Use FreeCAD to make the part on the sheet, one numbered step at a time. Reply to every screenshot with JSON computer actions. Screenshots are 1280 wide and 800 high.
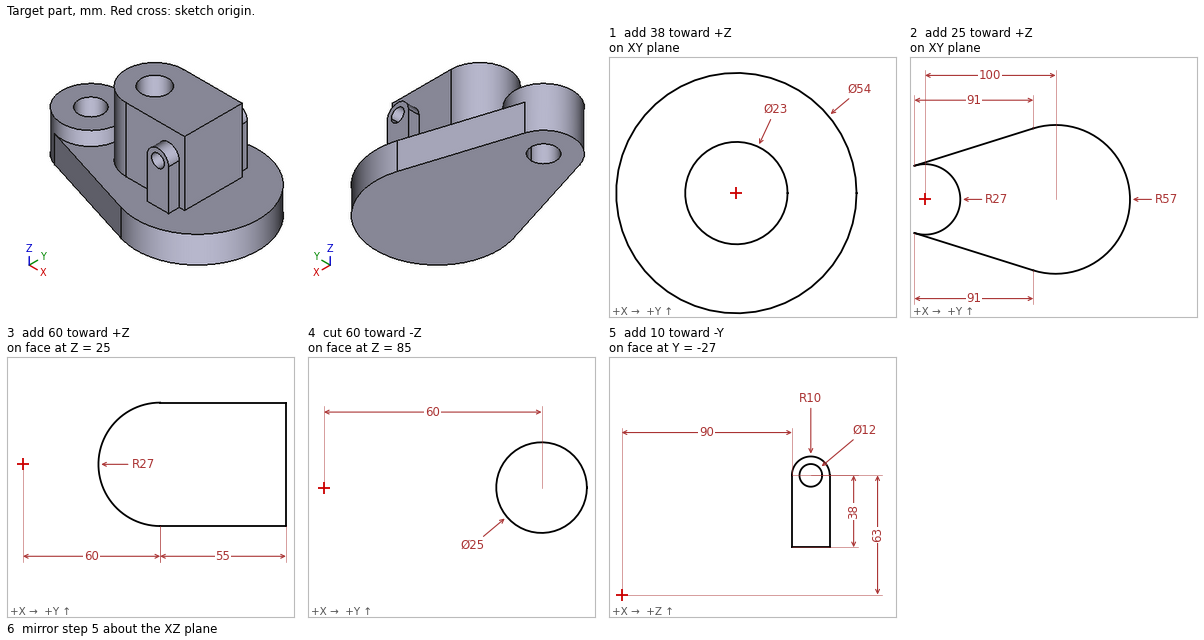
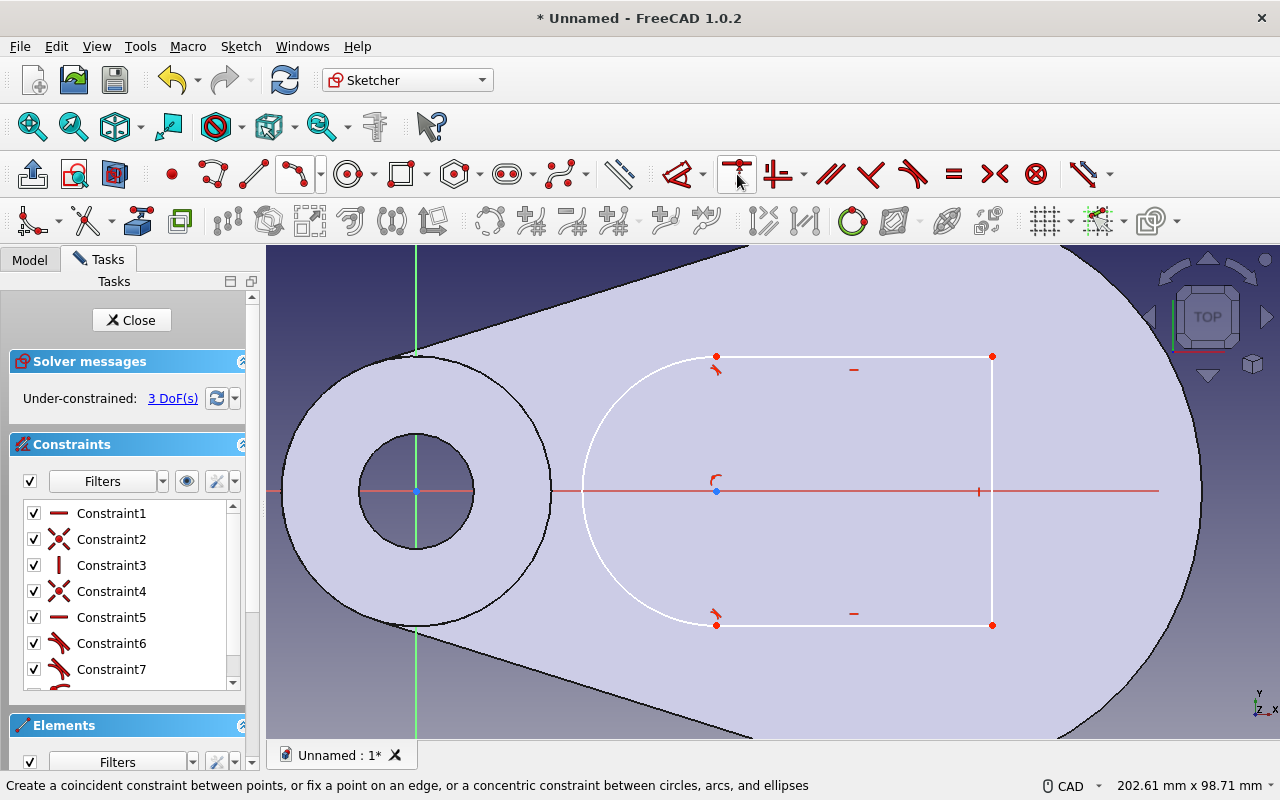
{"action": "left_click", "coordinate": [608, 412]}
{"action": "left_click", "coordinate": [582, 393]}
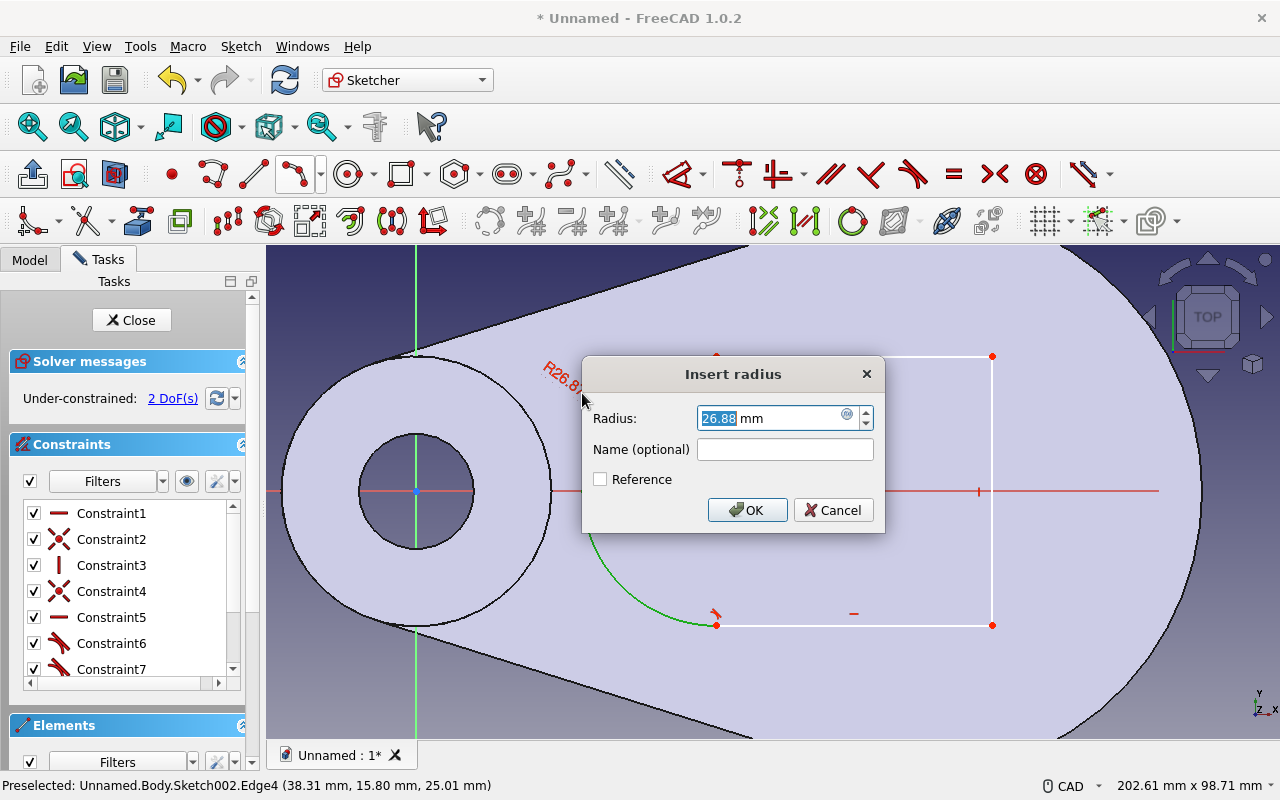
{"action": "type", "text": "27"}
{"action": "key", "text": "Return"}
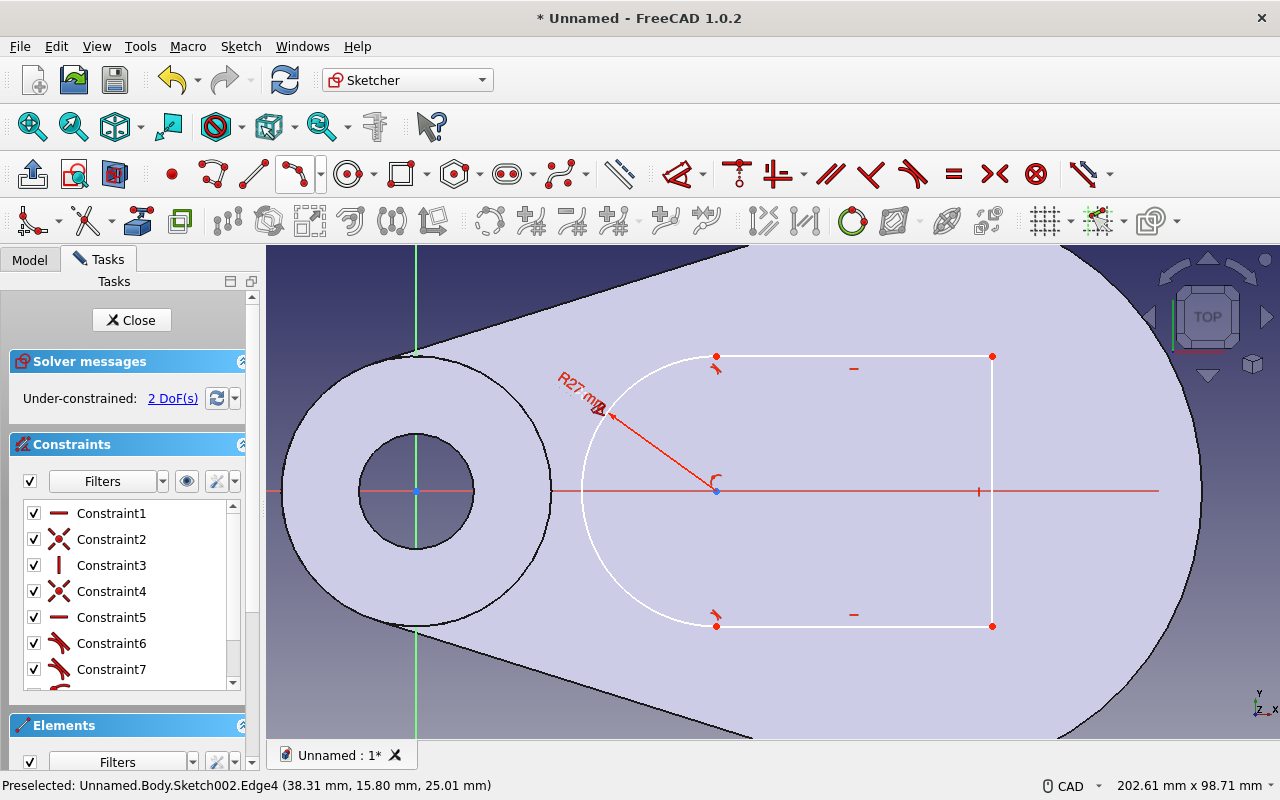
{"action": "left_click", "coordinate": [799, 627]}
{"action": "left_click", "coordinate": [854, 661]}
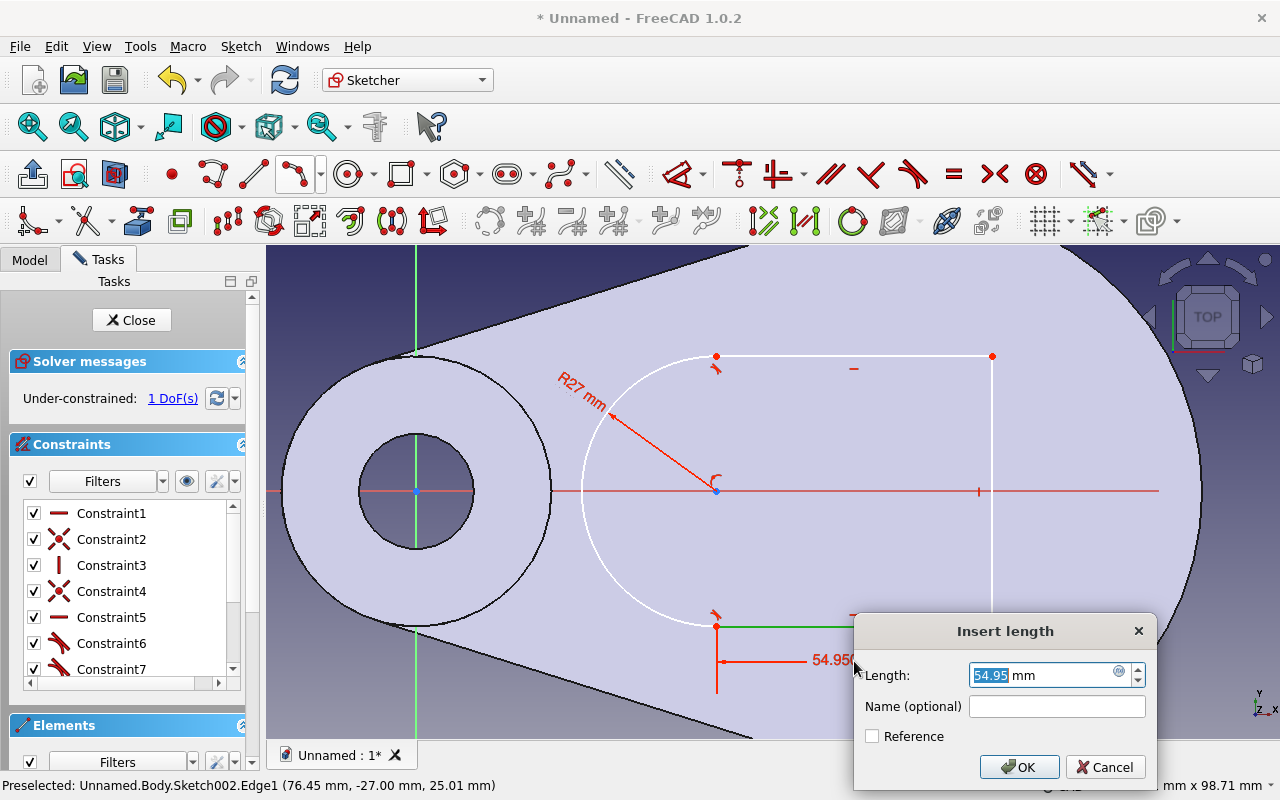
{"action": "type", "text": "55"}
{"action": "key", "text": "Return"}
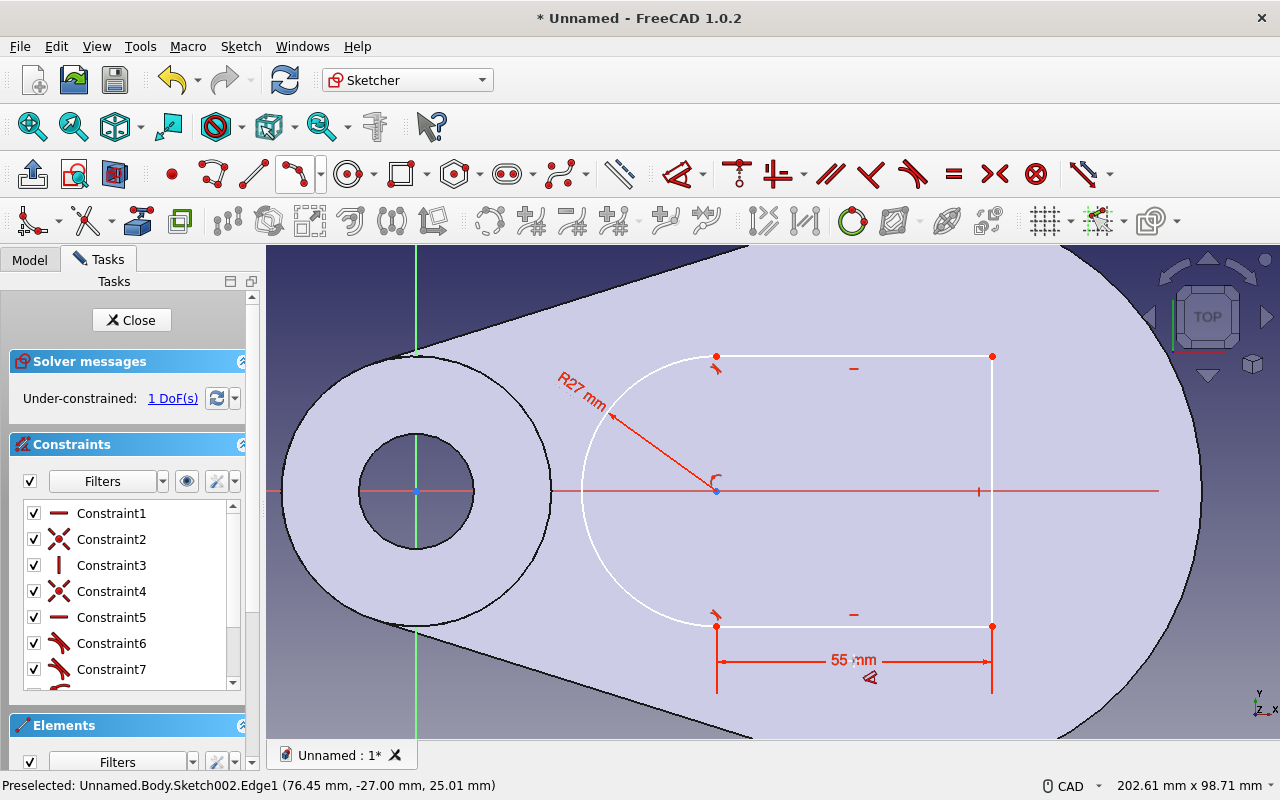
{"action": "left_click", "coordinate": [717, 627]}
{"action": "left_click", "coordinate": [567, 661]}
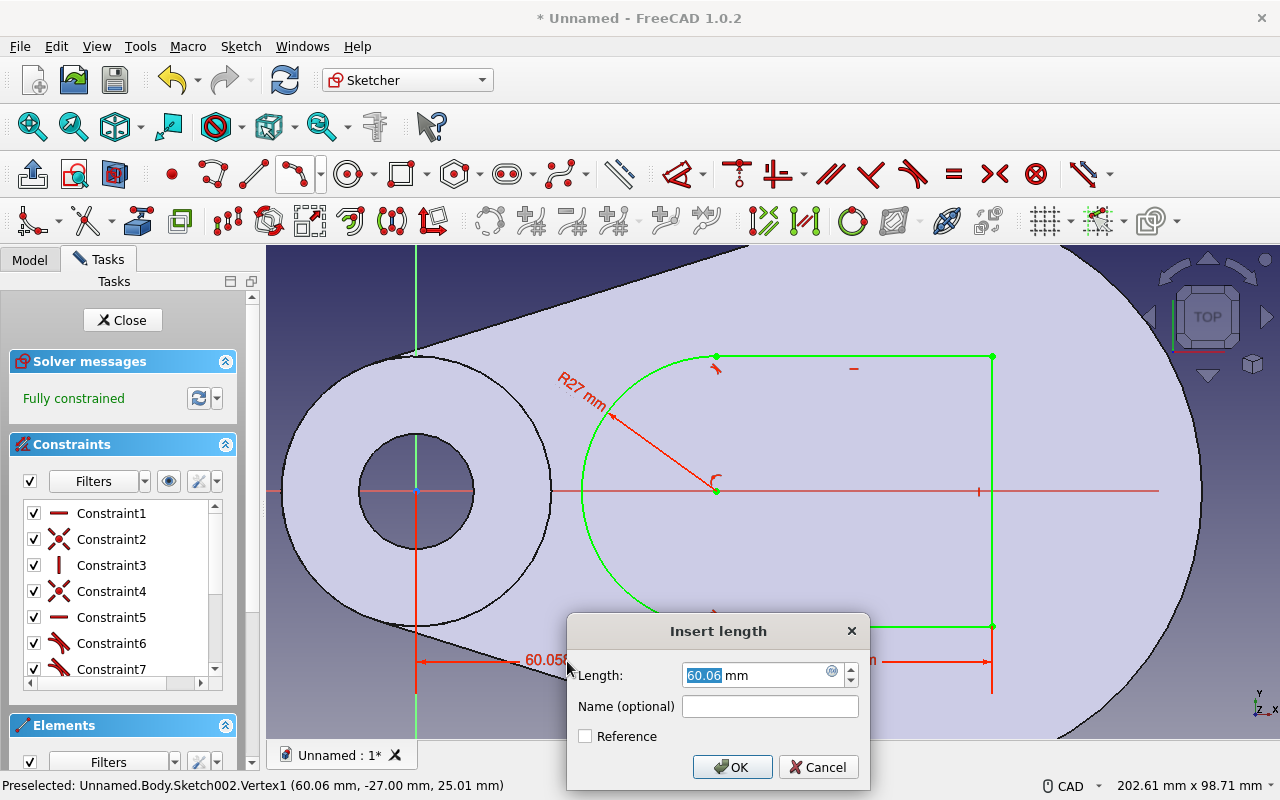
{"action": "type", "text": "60"}
{"action": "key", "text": "Return"}
{"action": "key", "text": "Escape"}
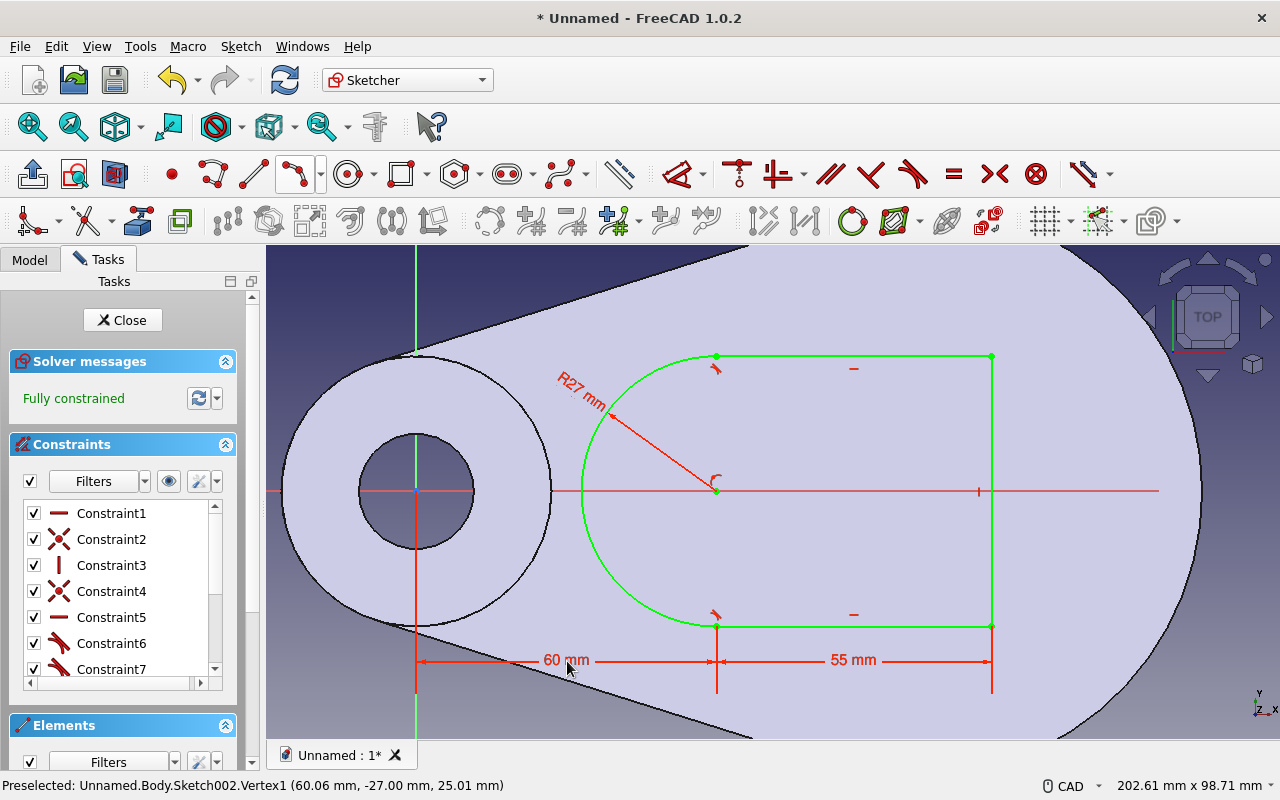
{"action": "left_click", "coordinate": [123, 320]}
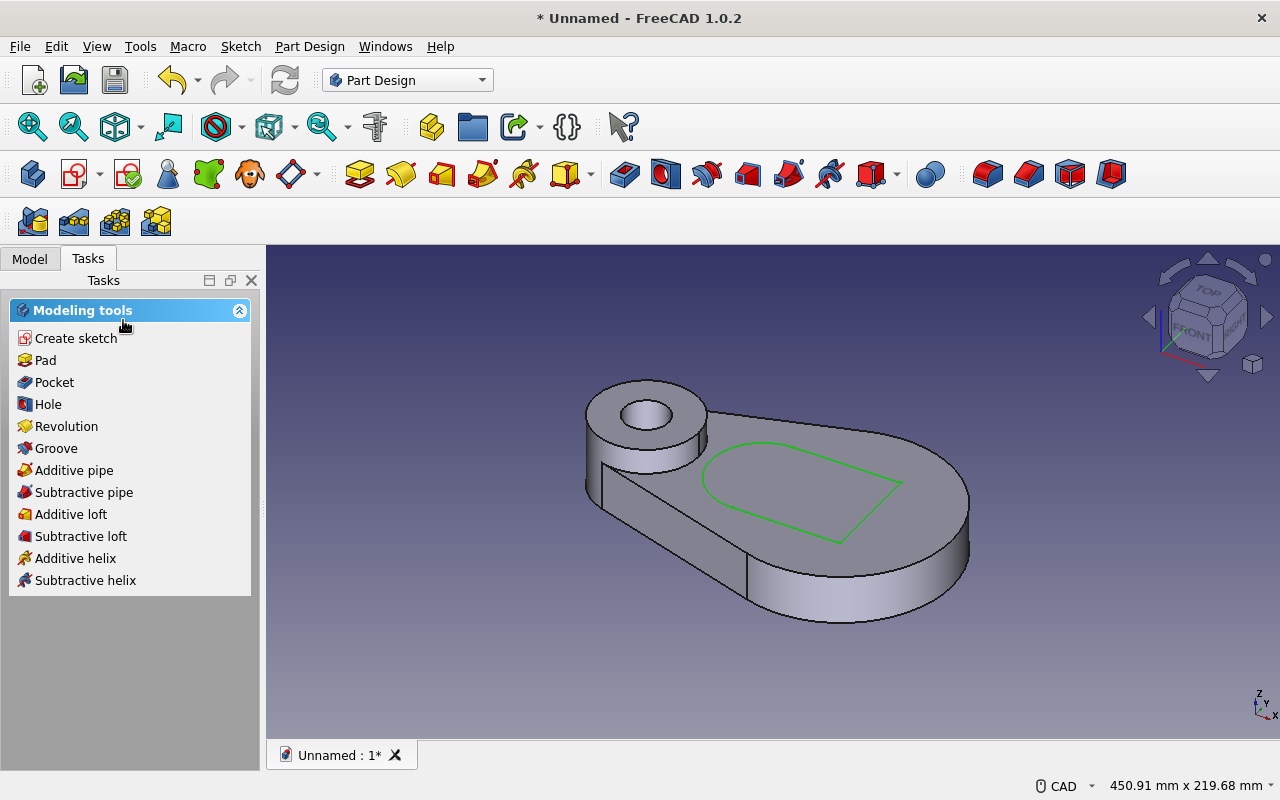
{"action": "left_click", "coordinate": [360, 174]}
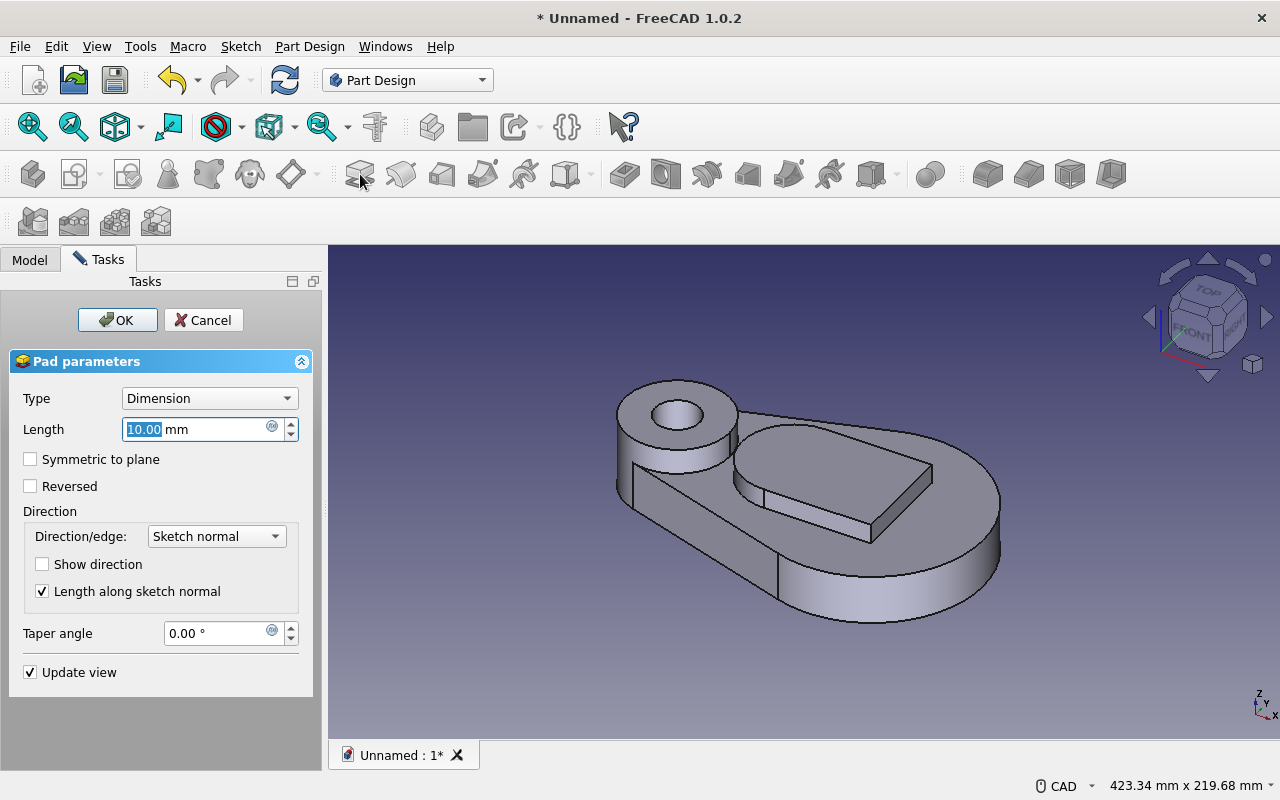
{"action": "type", "text": "60"}
{"action": "key", "text": "Tab"}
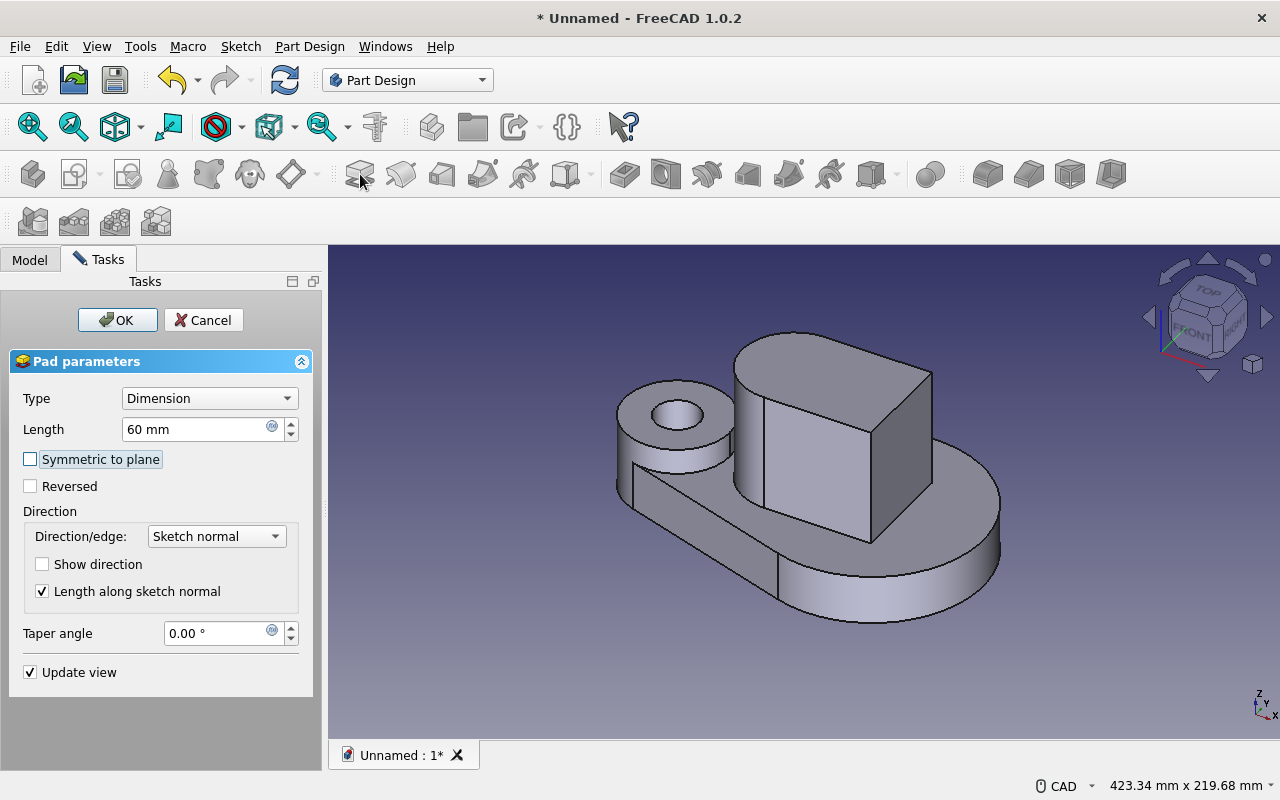
{"action": "left_click", "coordinate": [118, 320]}